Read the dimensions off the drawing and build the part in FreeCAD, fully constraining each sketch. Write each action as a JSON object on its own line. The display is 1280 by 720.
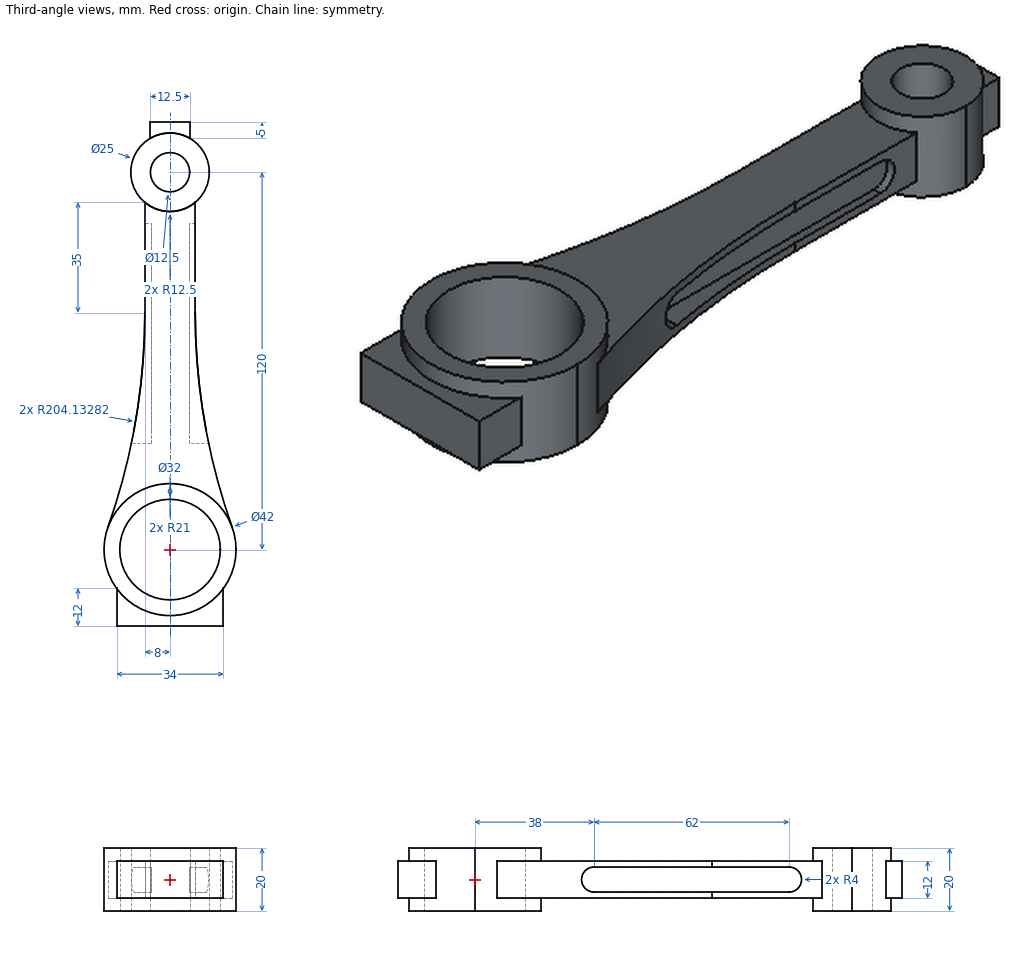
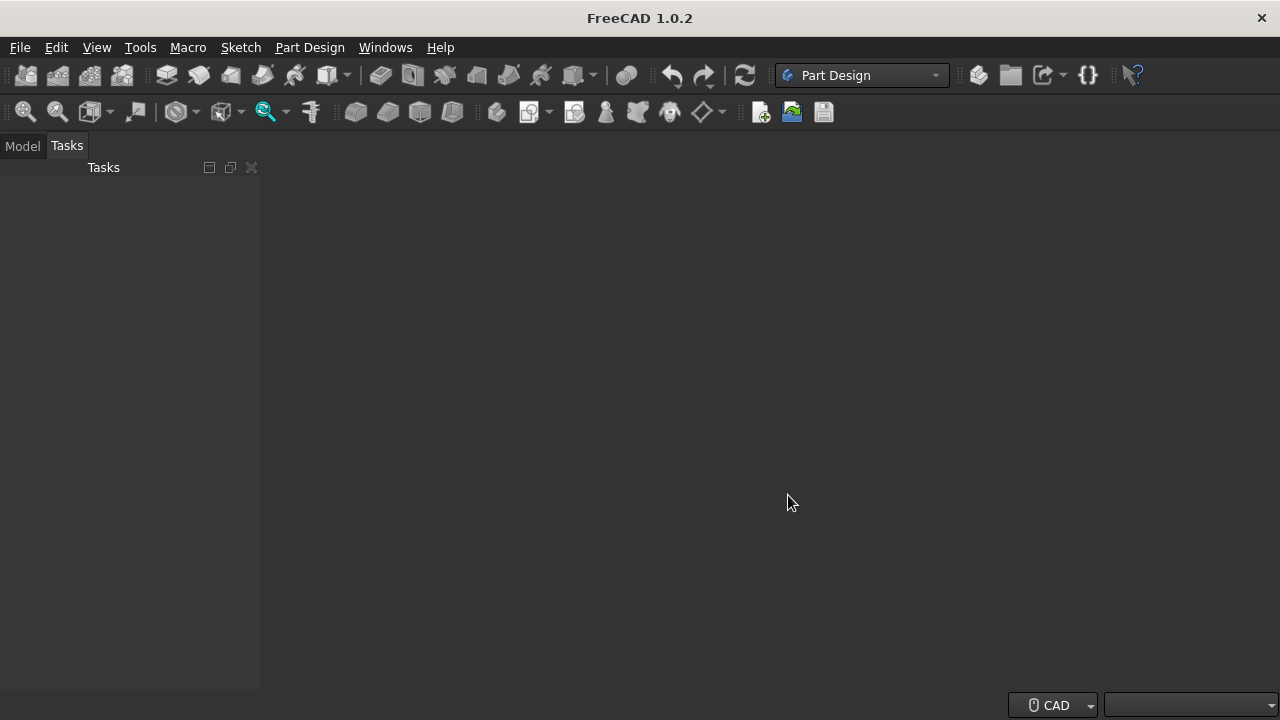
{"action": "key", "text": "ctrl+n"}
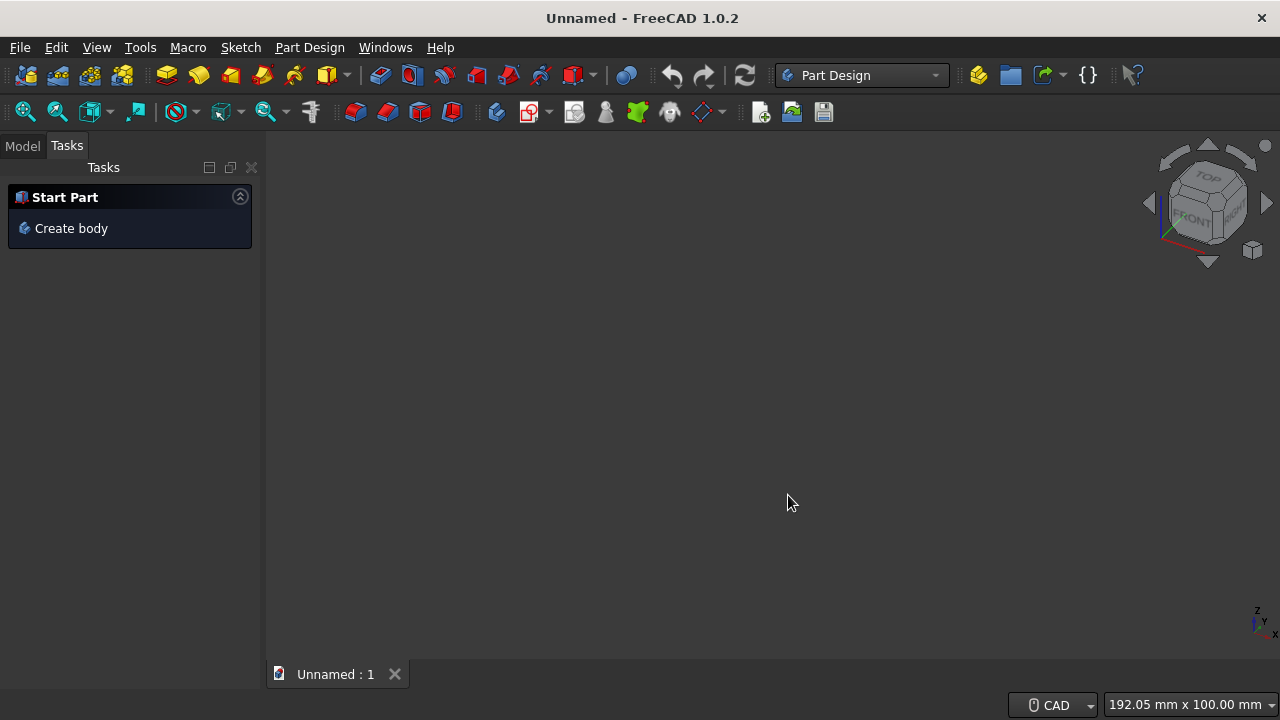
{"action": "left_click", "coordinate": [530, 112]}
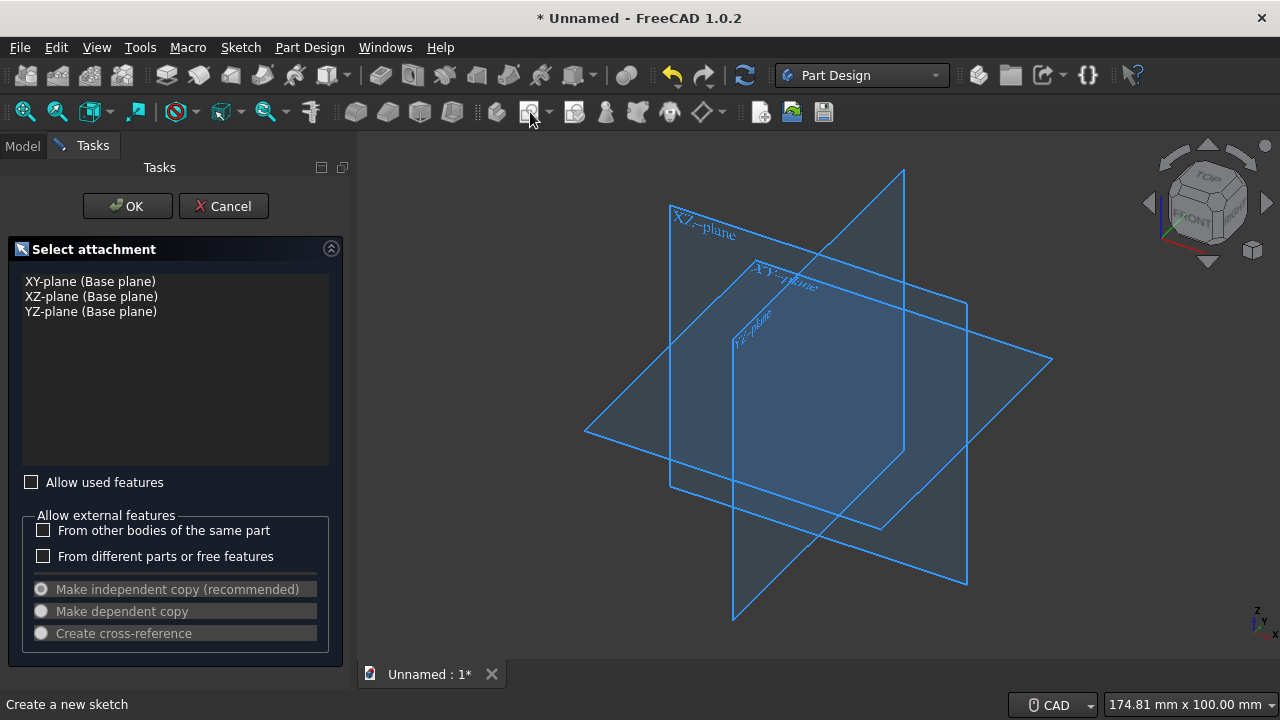
{"action": "left_click", "coordinate": [82, 282]}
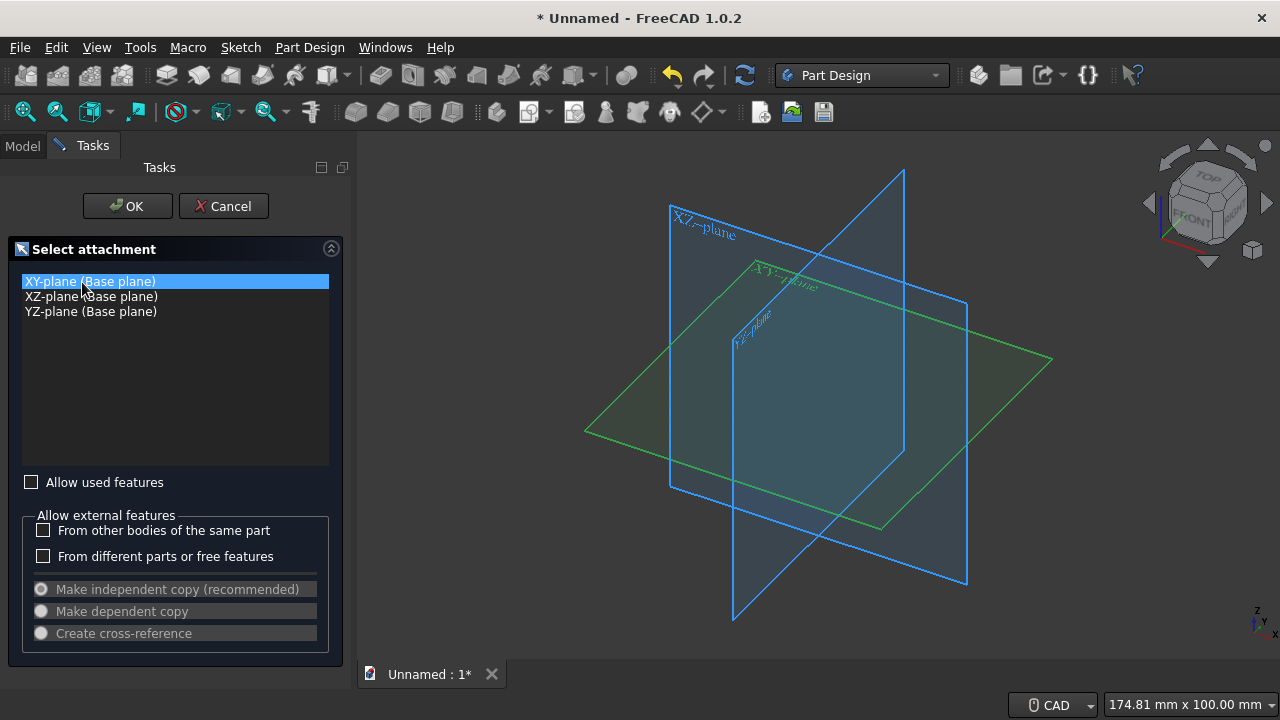
{"action": "left_click", "coordinate": [128, 206]}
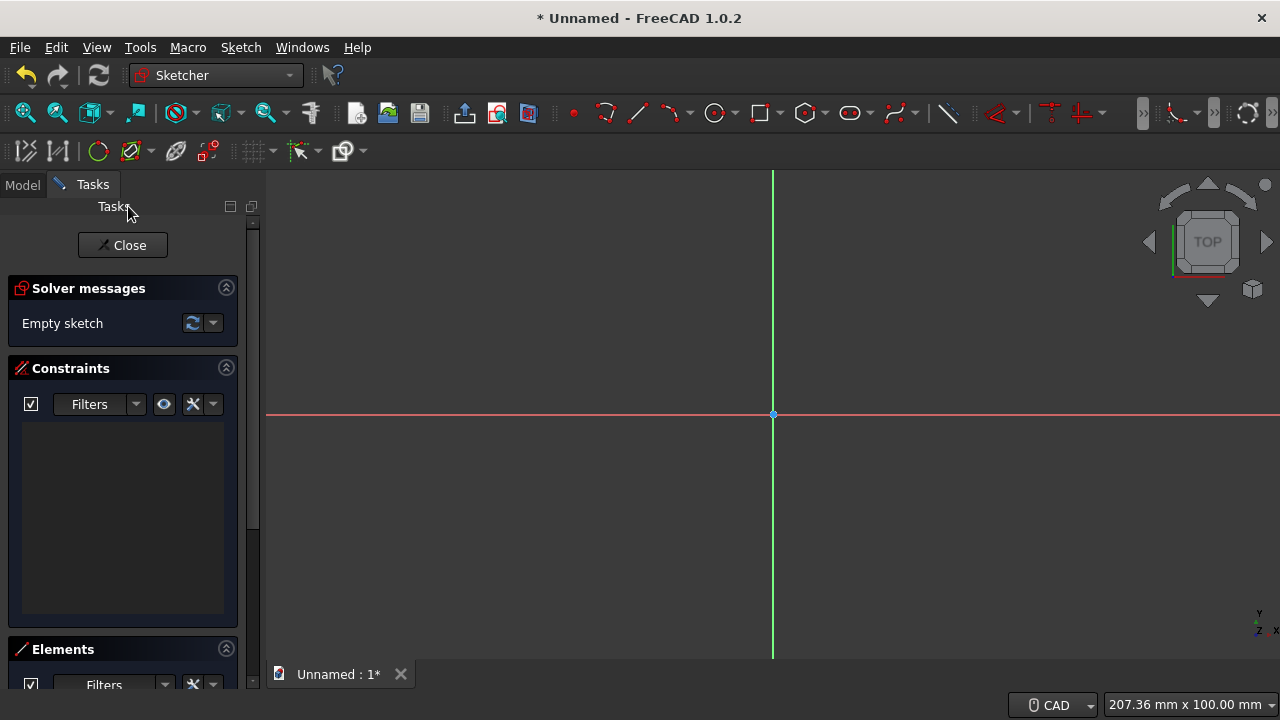
{"action": "scroll", "coordinate": [704, 414], "scroll_direction": "down", "scroll_amount": 5}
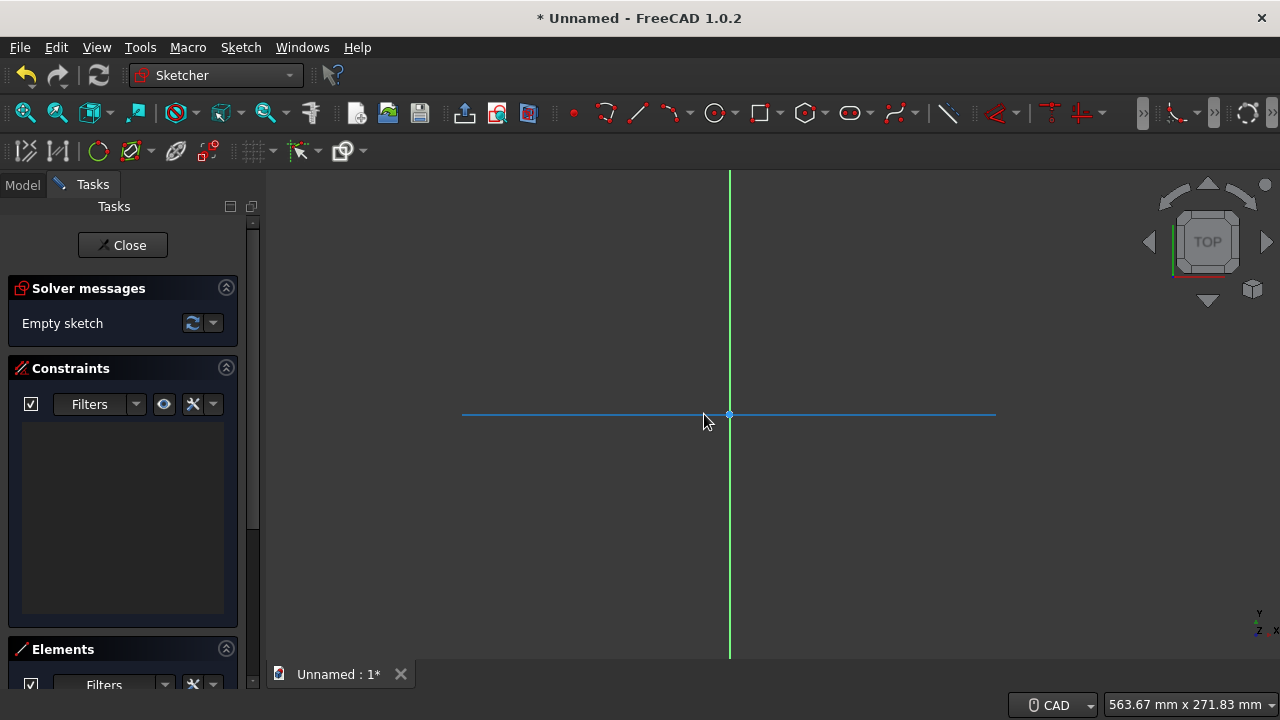
{"action": "scroll", "coordinate": [704, 414], "scroll_direction": "down", "scroll_amount": 5}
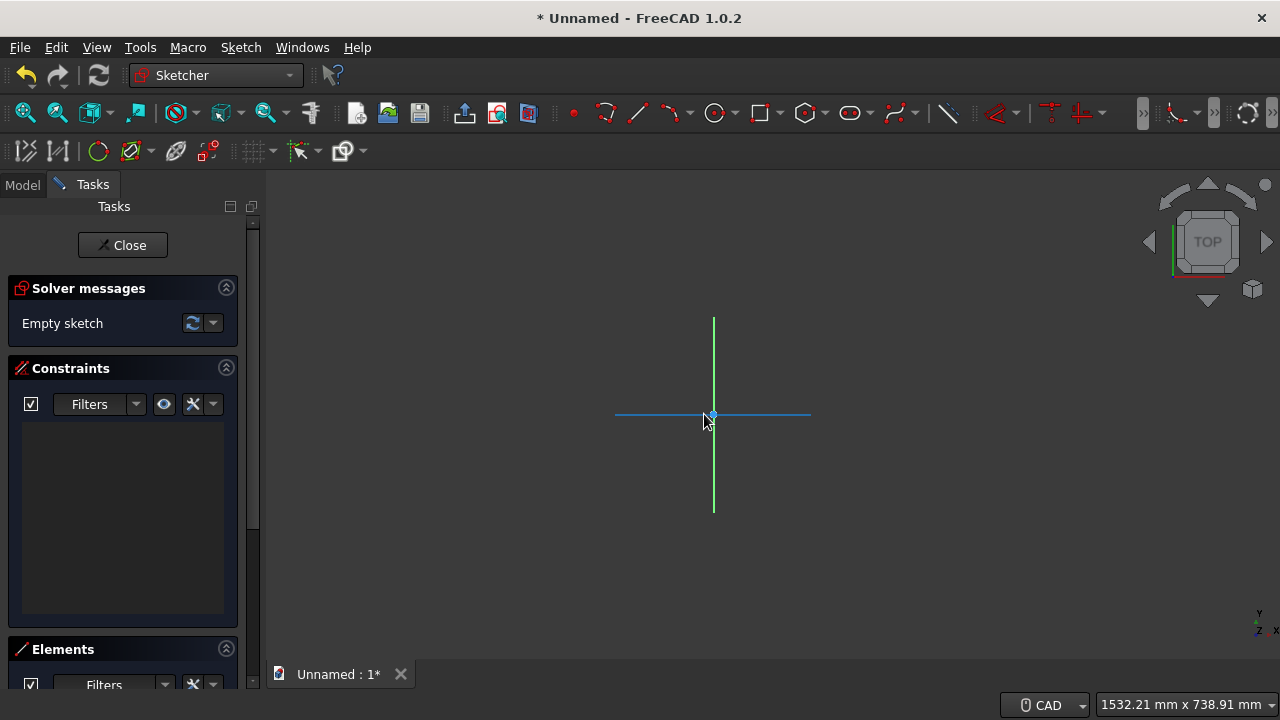
{"action": "scroll", "coordinate": [714, 331], "scroll_direction": "up", "scroll_amount": 15}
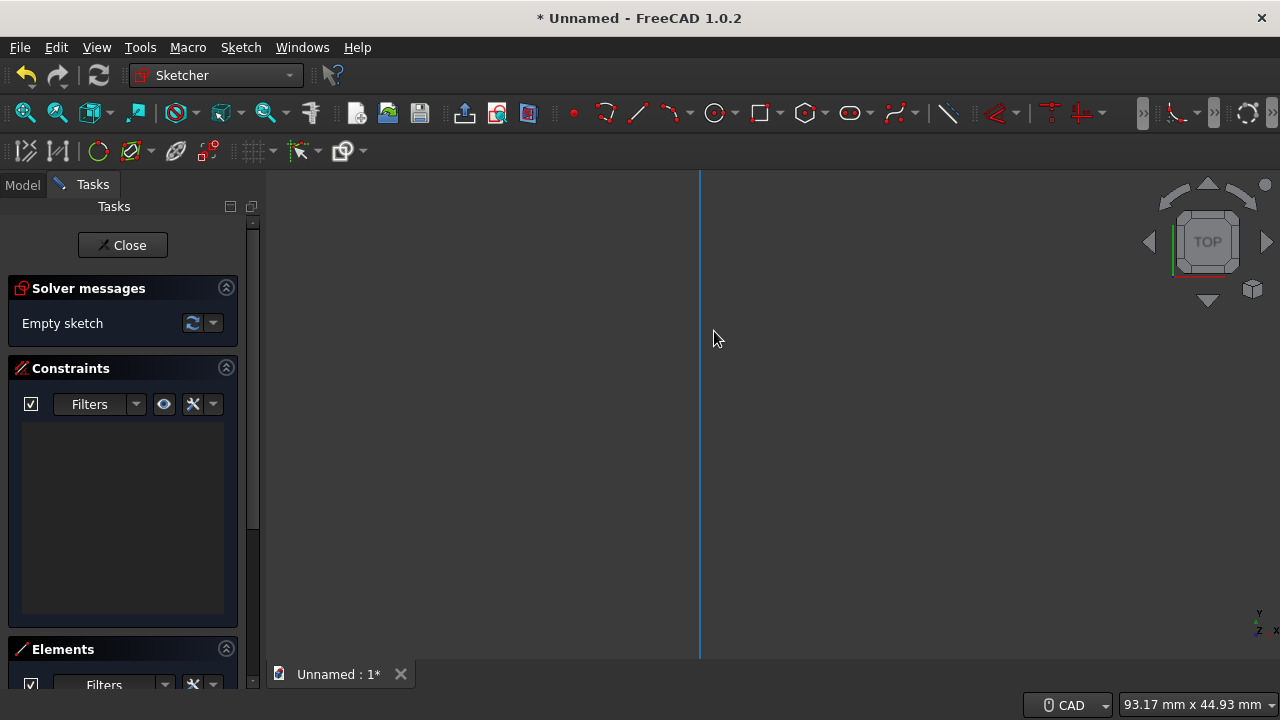
{"action": "key", "text": "g c"}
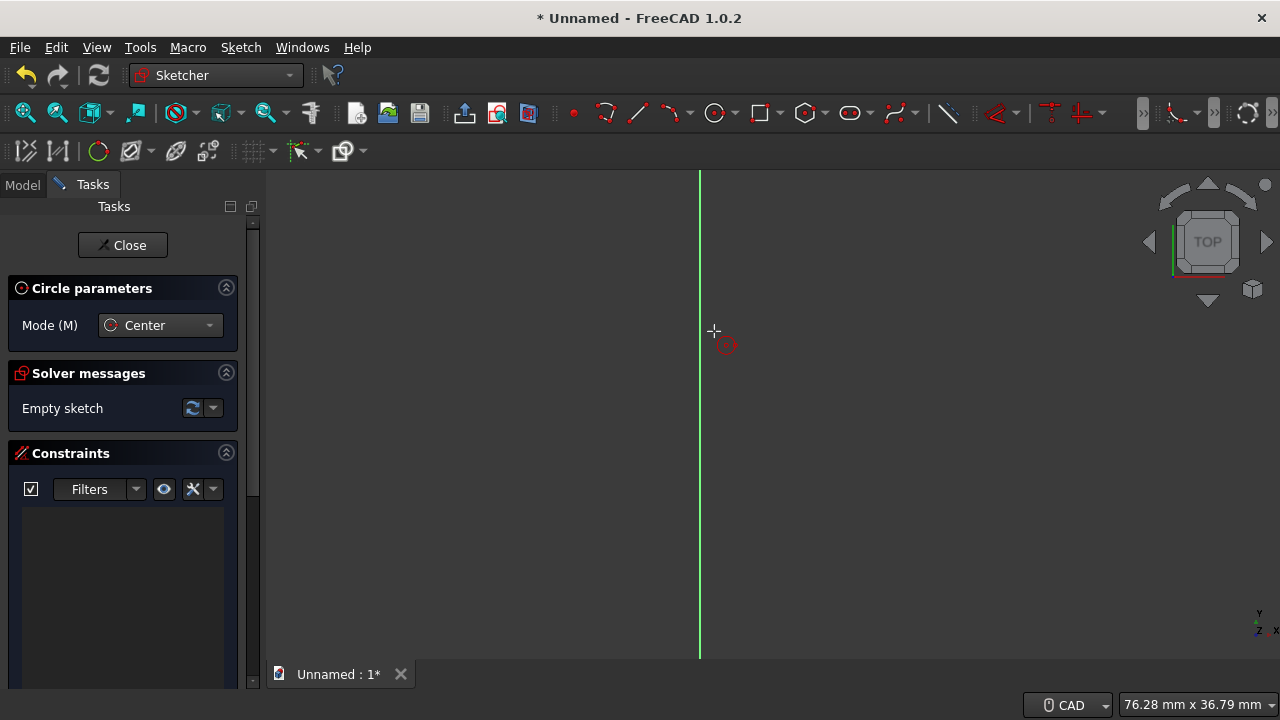
{"action": "left_click", "coordinate": [700, 407]}
{"action": "left_click", "coordinate": [817, 289]}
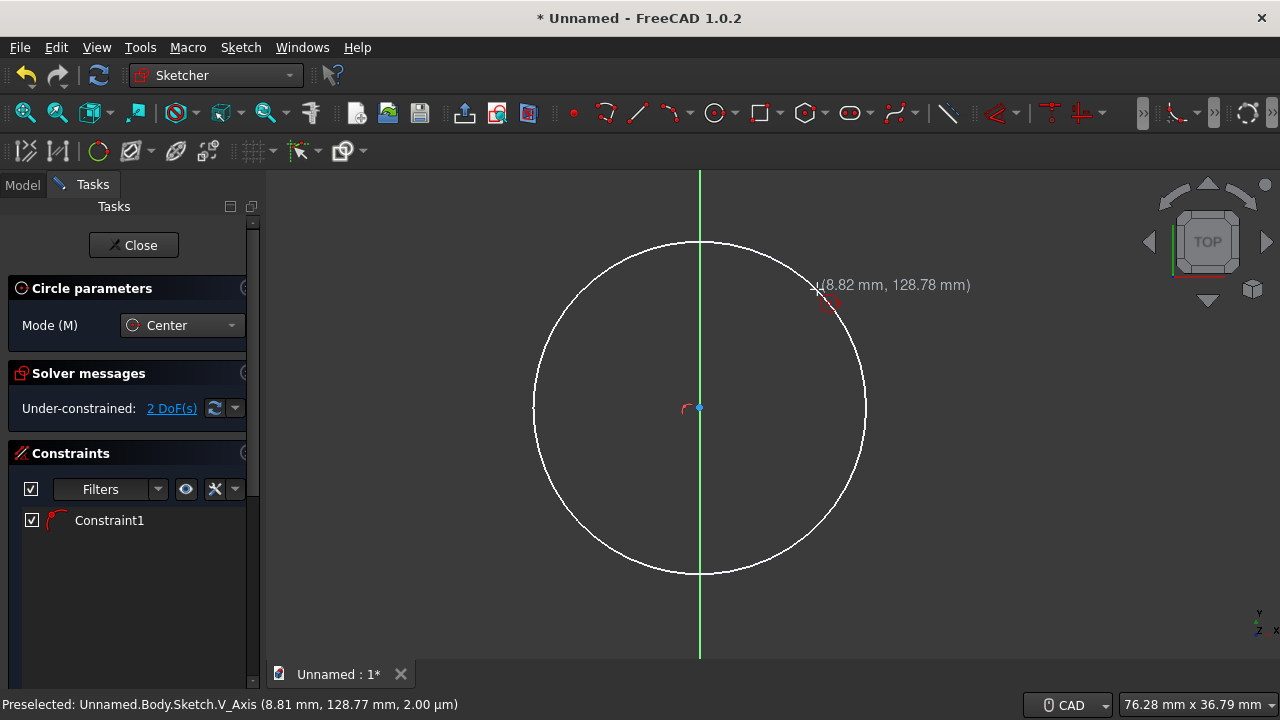
{"action": "left_click", "coordinate": [700, 408]}
{"action": "left_click", "coordinate": [759, 348]}
{"action": "key", "text": "Escape"}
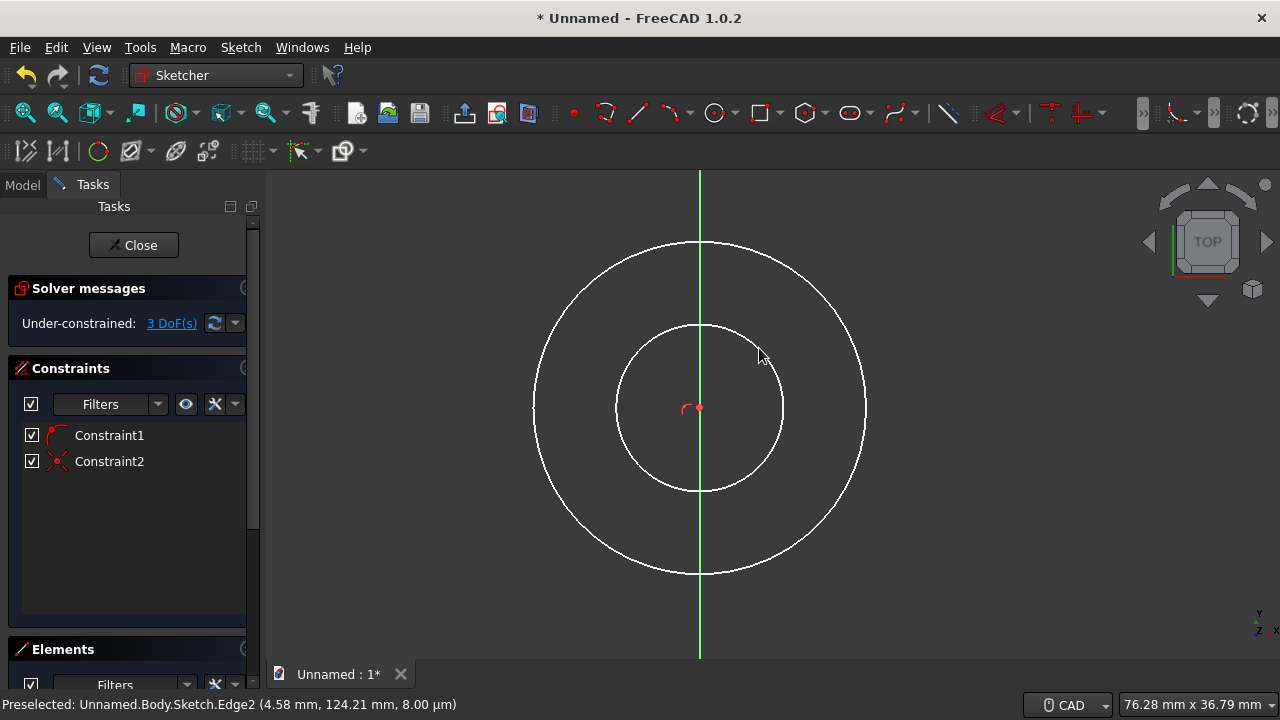
{"action": "left_click", "coordinate": [996, 114]}